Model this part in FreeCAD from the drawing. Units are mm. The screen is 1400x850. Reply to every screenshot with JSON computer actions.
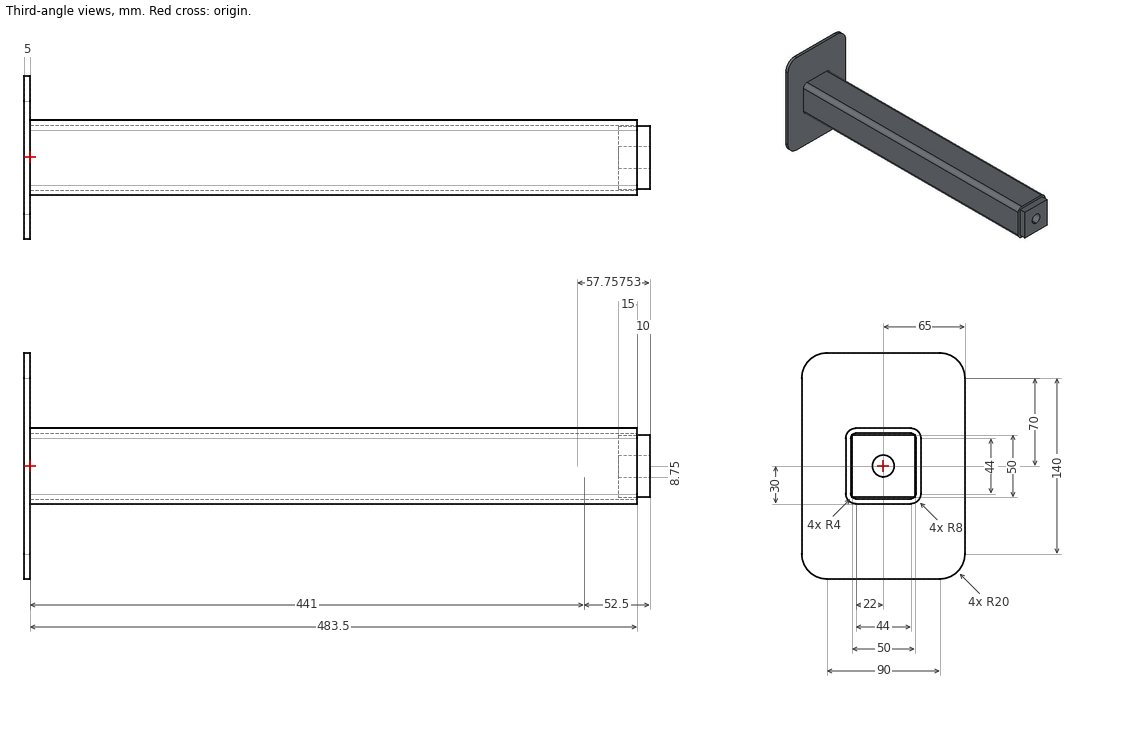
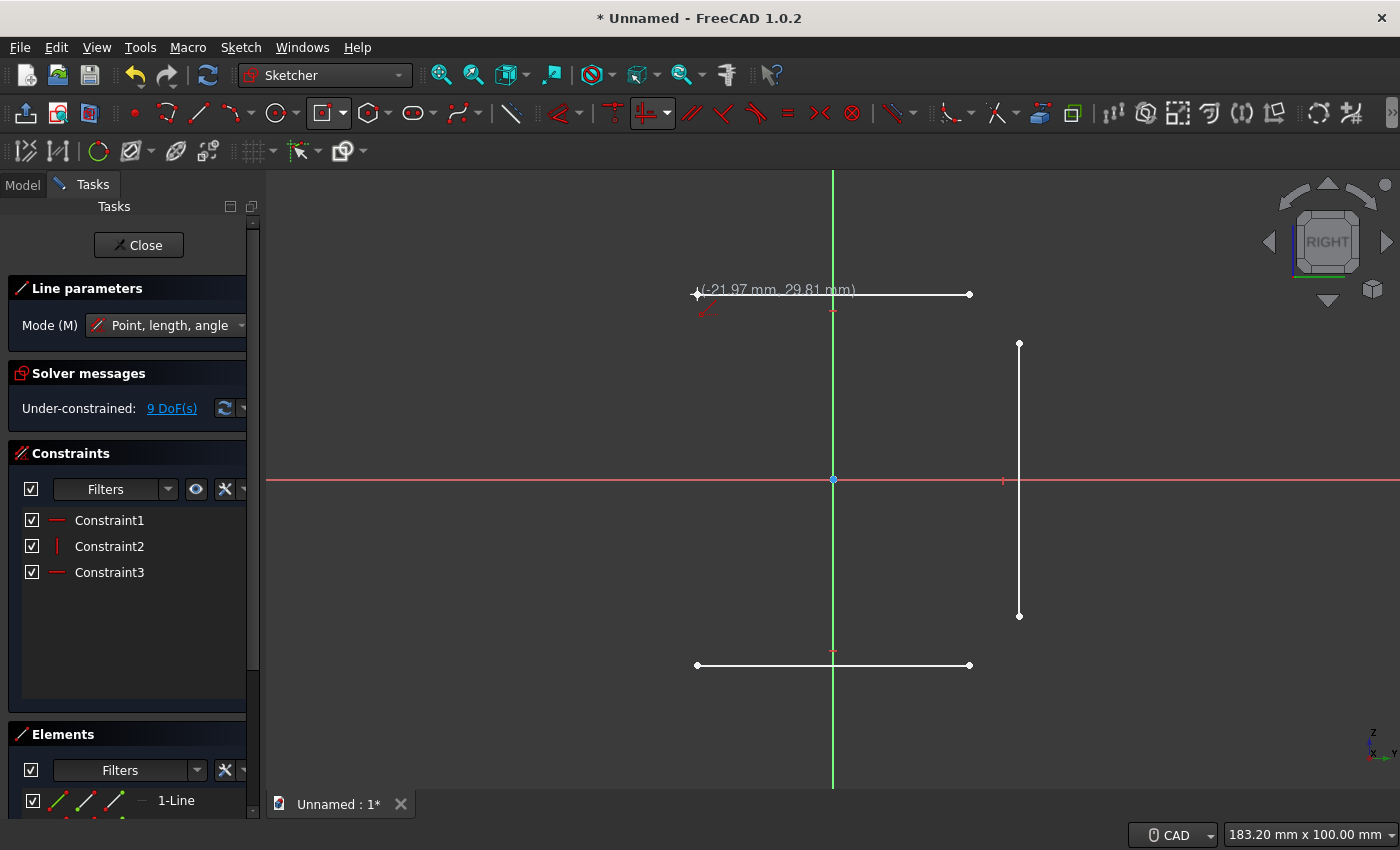
{"action": "left_click", "coordinate": [647, 343]}
{"action": "left_click", "coordinate": [647, 616]}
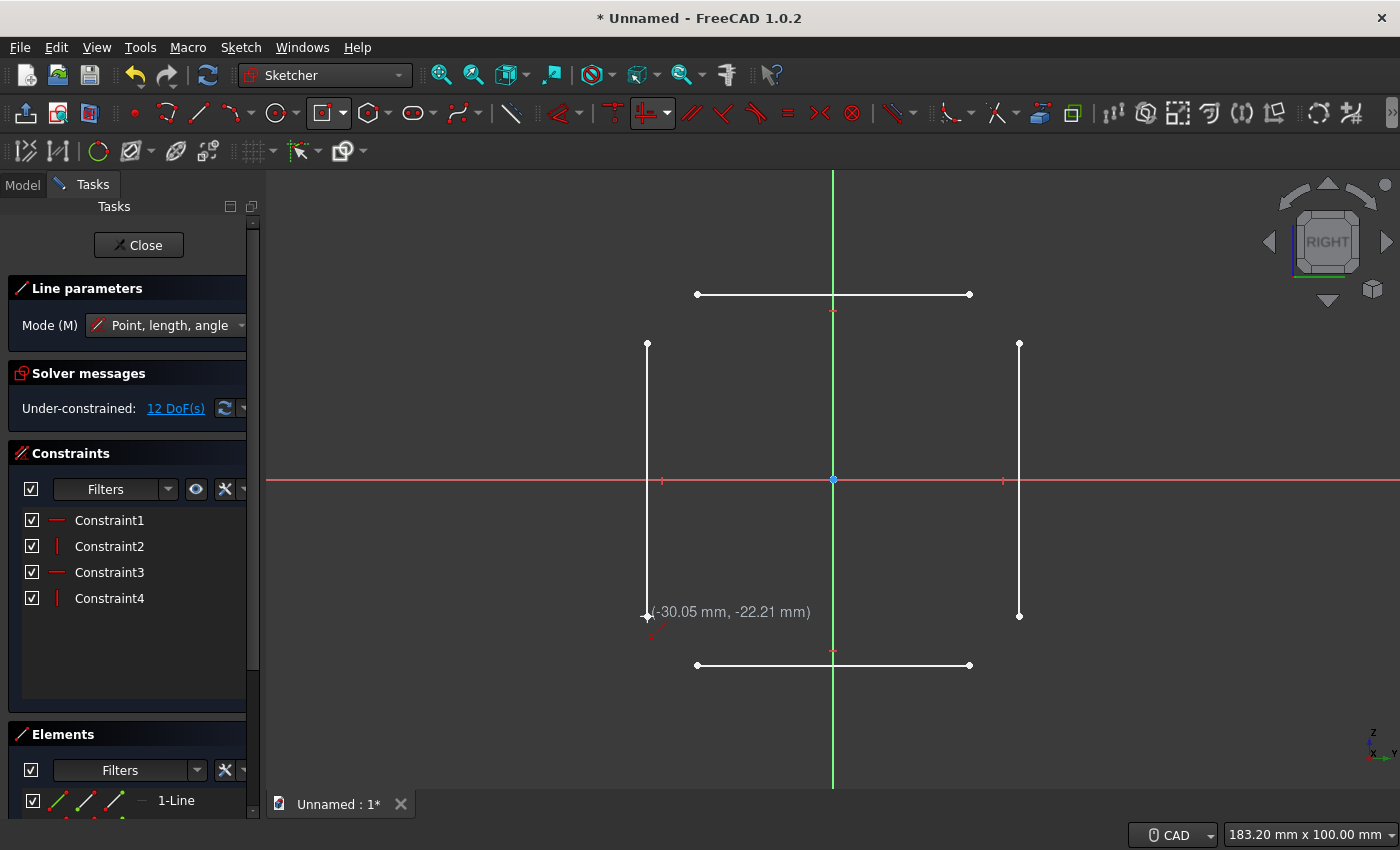
{"action": "key", "text": "g 3 a"}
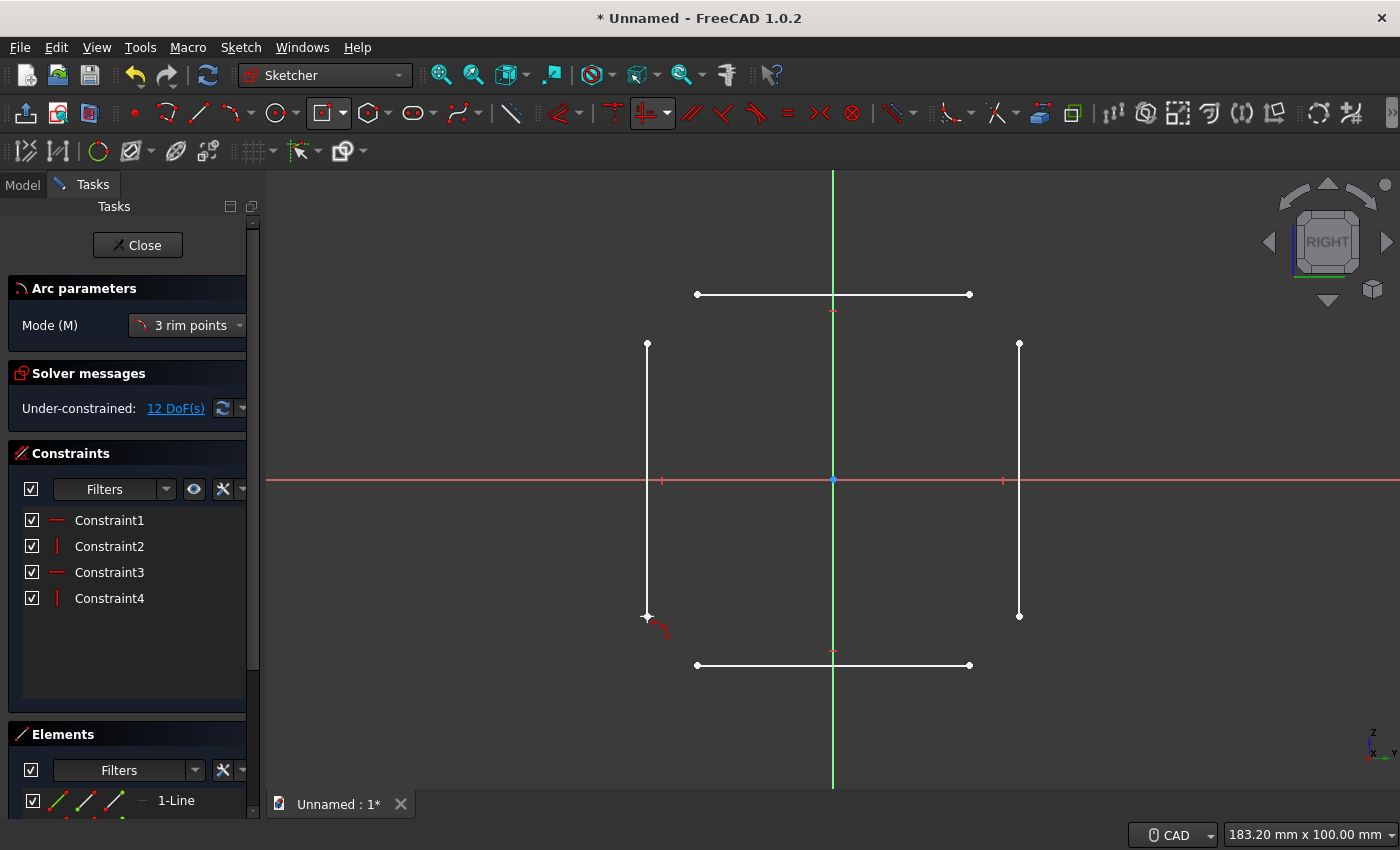
{"action": "left_click", "coordinate": [969, 666]}
{"action": "left_click", "coordinate": [1019, 617]}
{"action": "left_click", "coordinate": [1004, 651]}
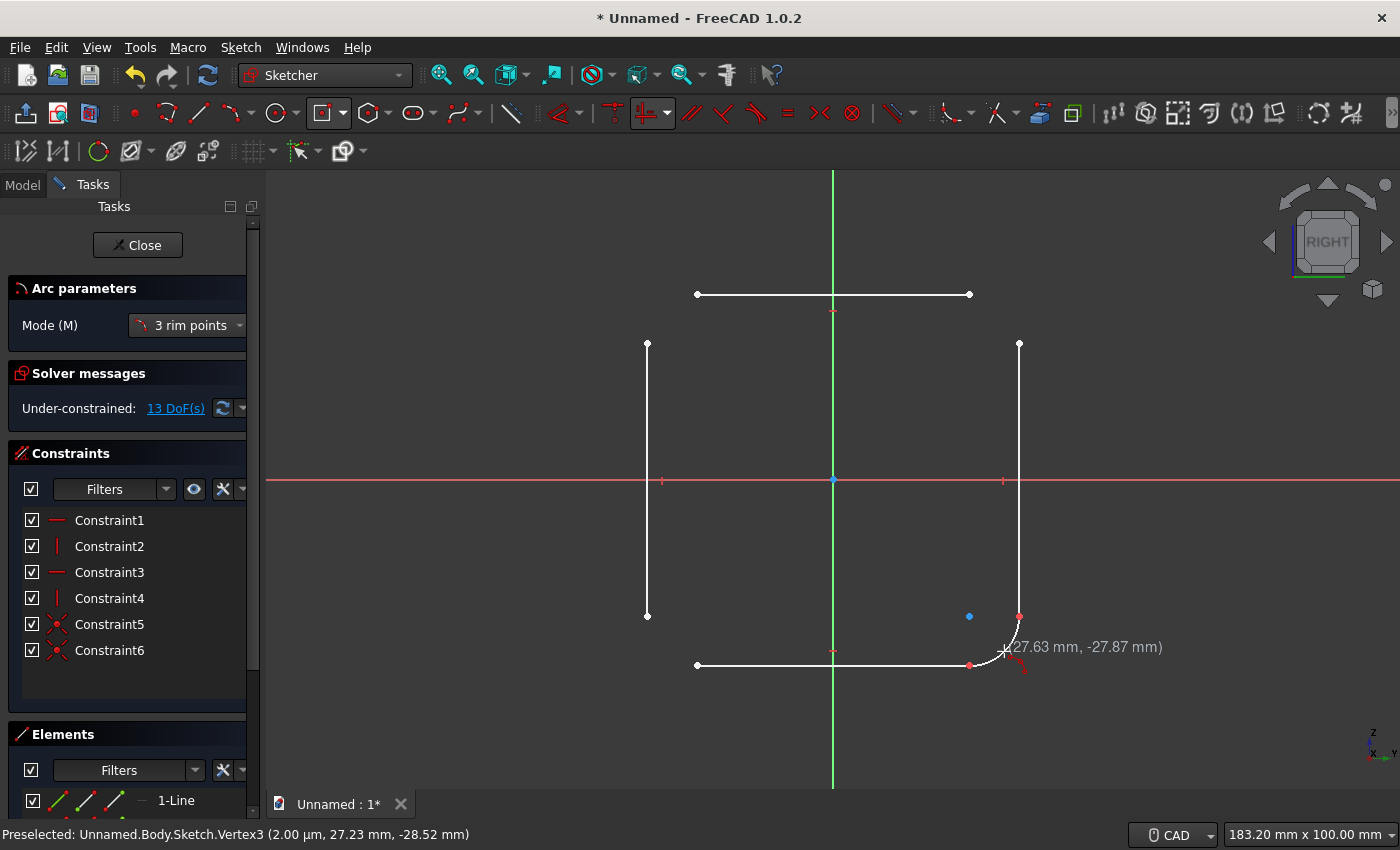
{"action": "left_click", "coordinate": [1019, 344]}
{"action": "left_click", "coordinate": [969, 295]}
{"action": "left_click", "coordinate": [1004, 308]}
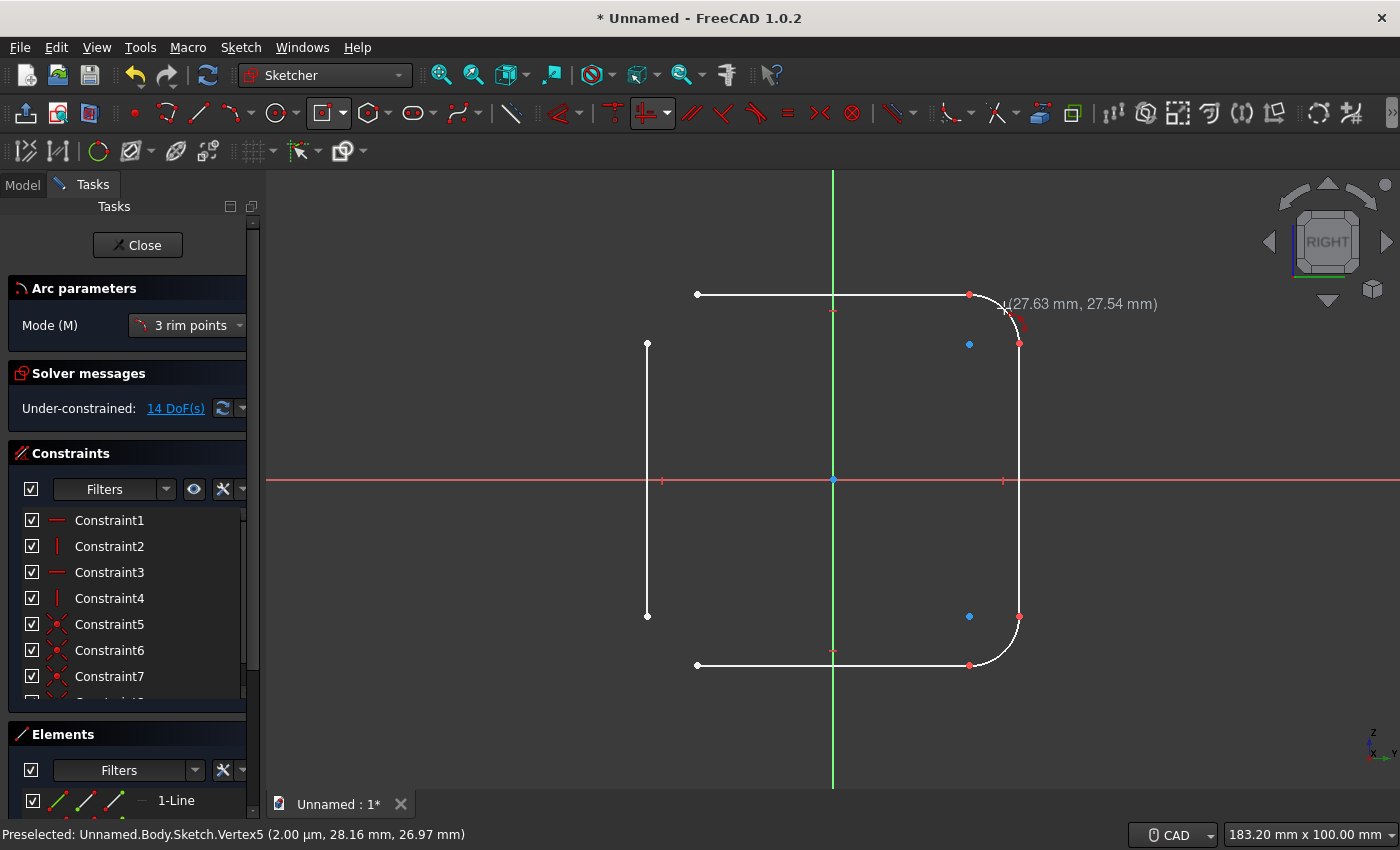
{"action": "left_click", "coordinate": [697, 295]}
{"action": "left_click", "coordinate": [647, 344]}
{"action": "left_click", "coordinate": [662, 308]}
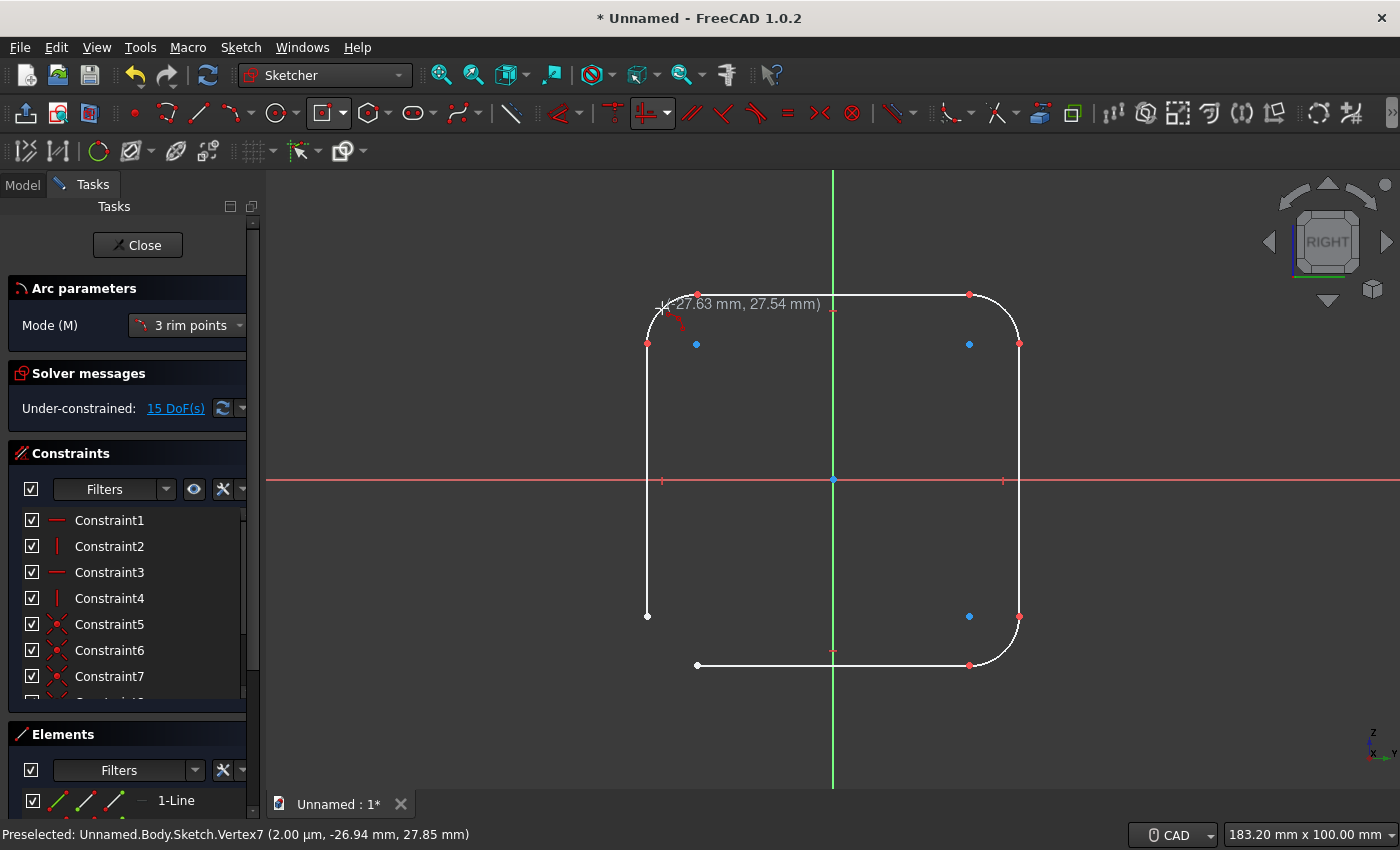
{"action": "left_click", "coordinate": [647, 617]}
{"action": "left_click", "coordinate": [697, 666]}
{"action": "left_click", "coordinate": [662, 651]}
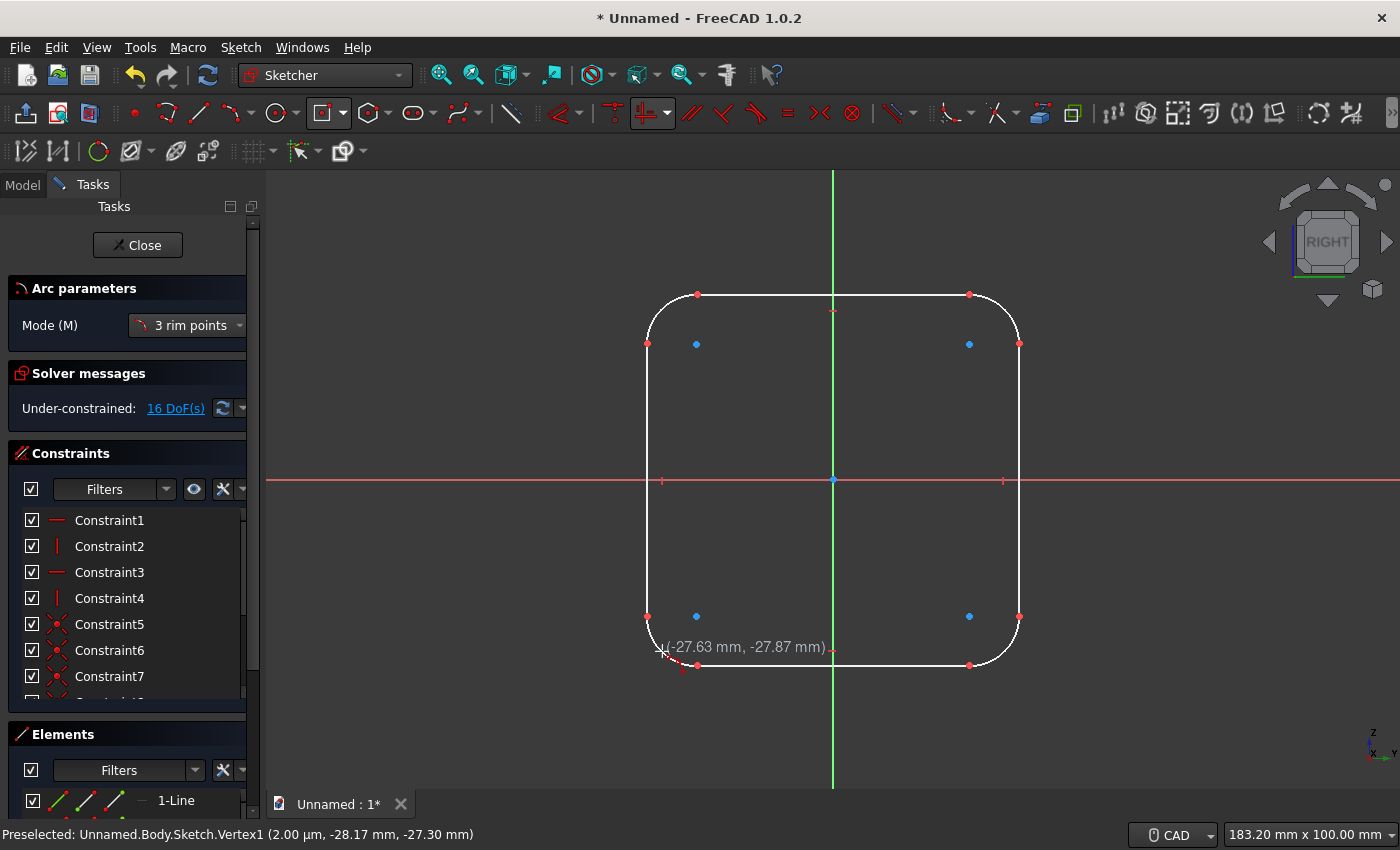
{"action": "key", "text": "g l"}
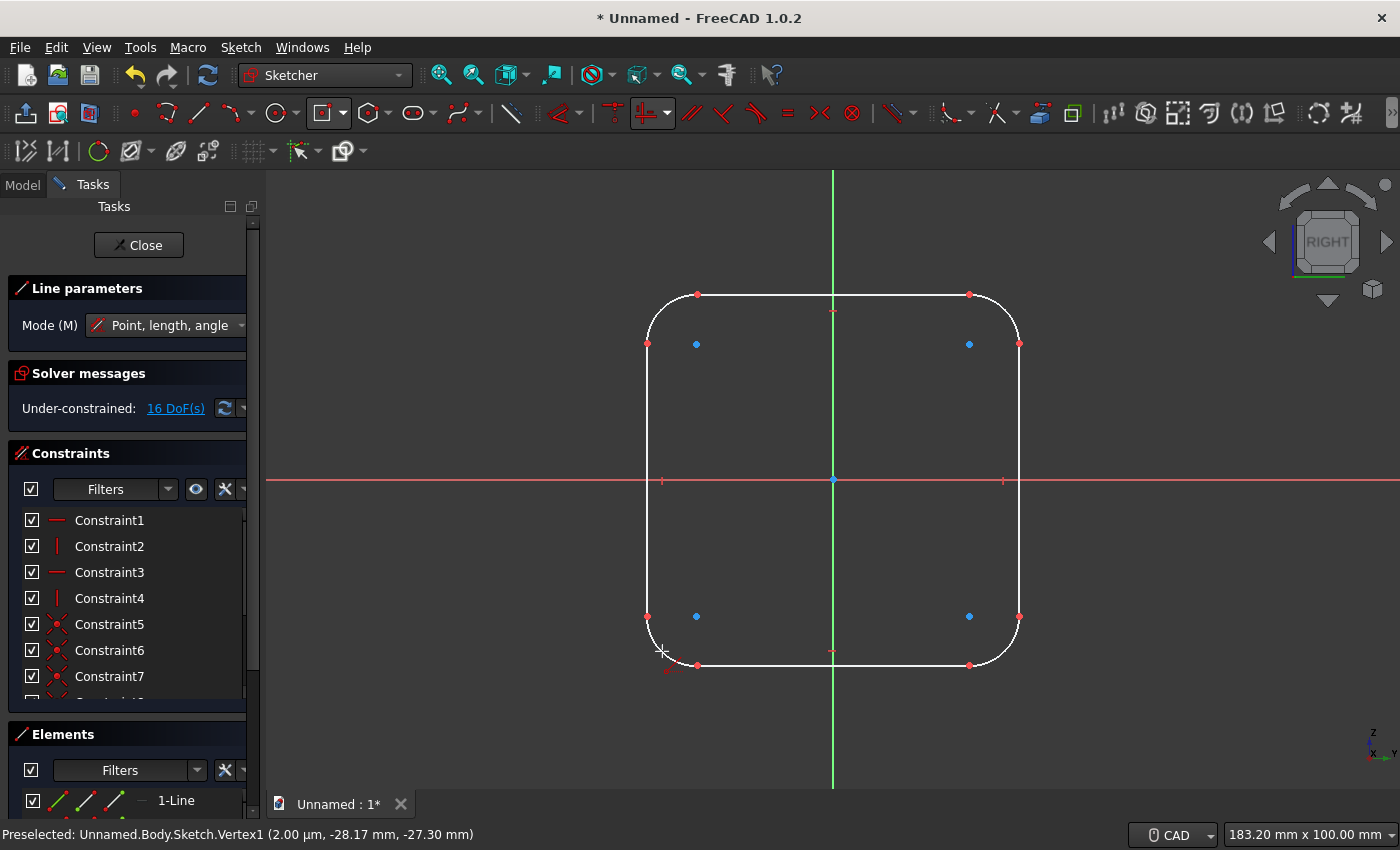
{"action": "left_click", "coordinate": [969, 640]}
{"action": "left_click", "coordinate": [697, 640]}